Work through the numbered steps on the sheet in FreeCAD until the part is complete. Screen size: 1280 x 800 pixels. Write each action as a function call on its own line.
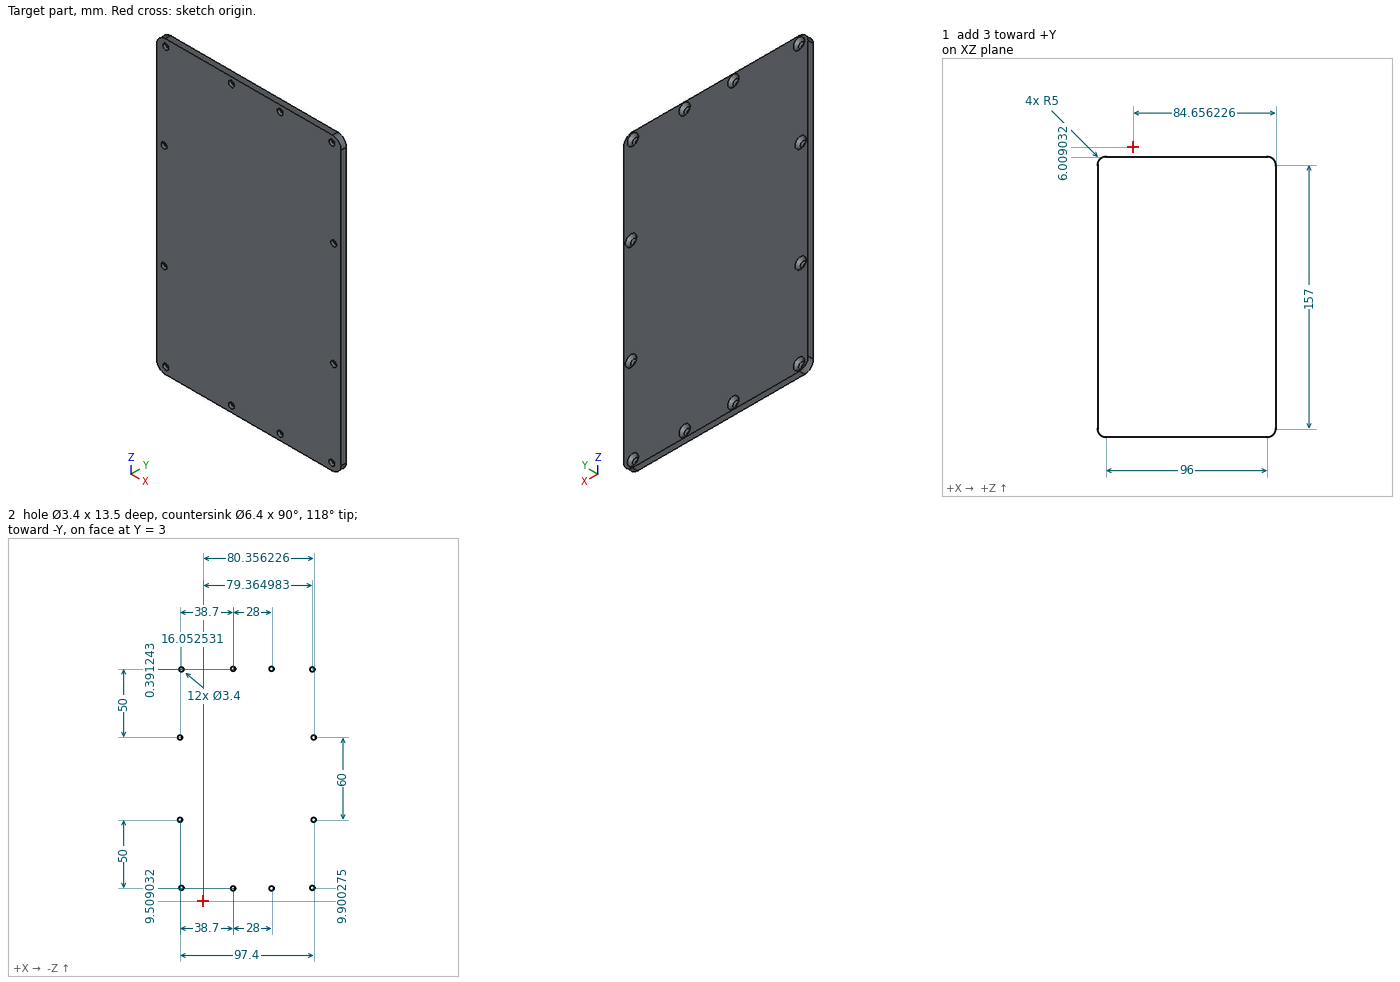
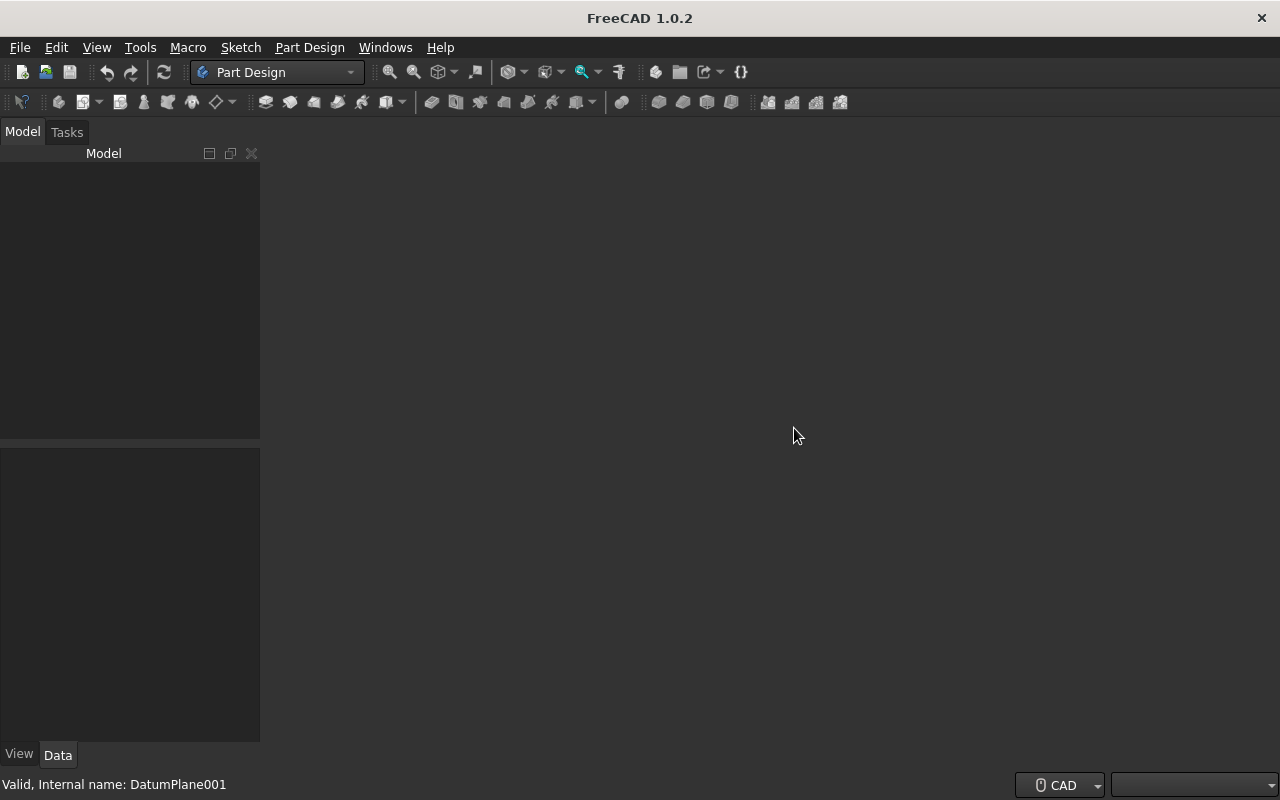
click(22, 72)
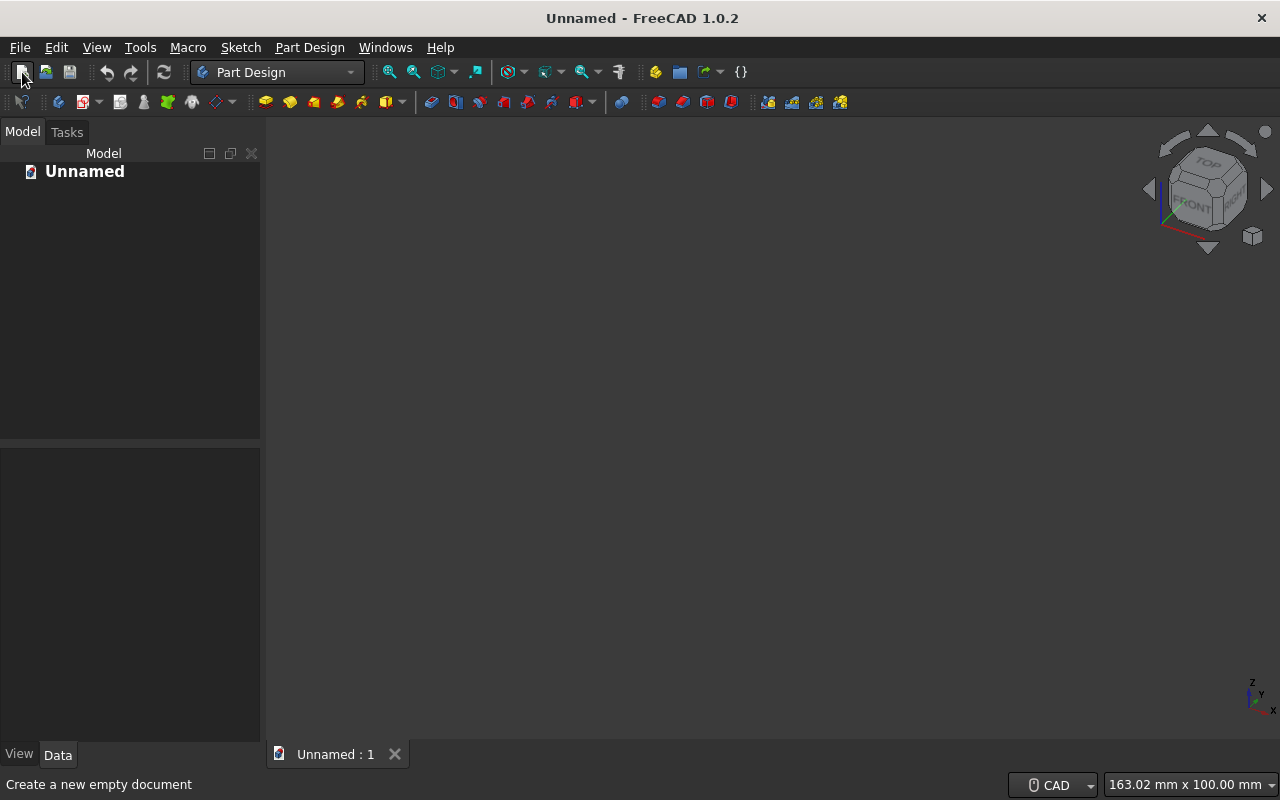
click(84, 102)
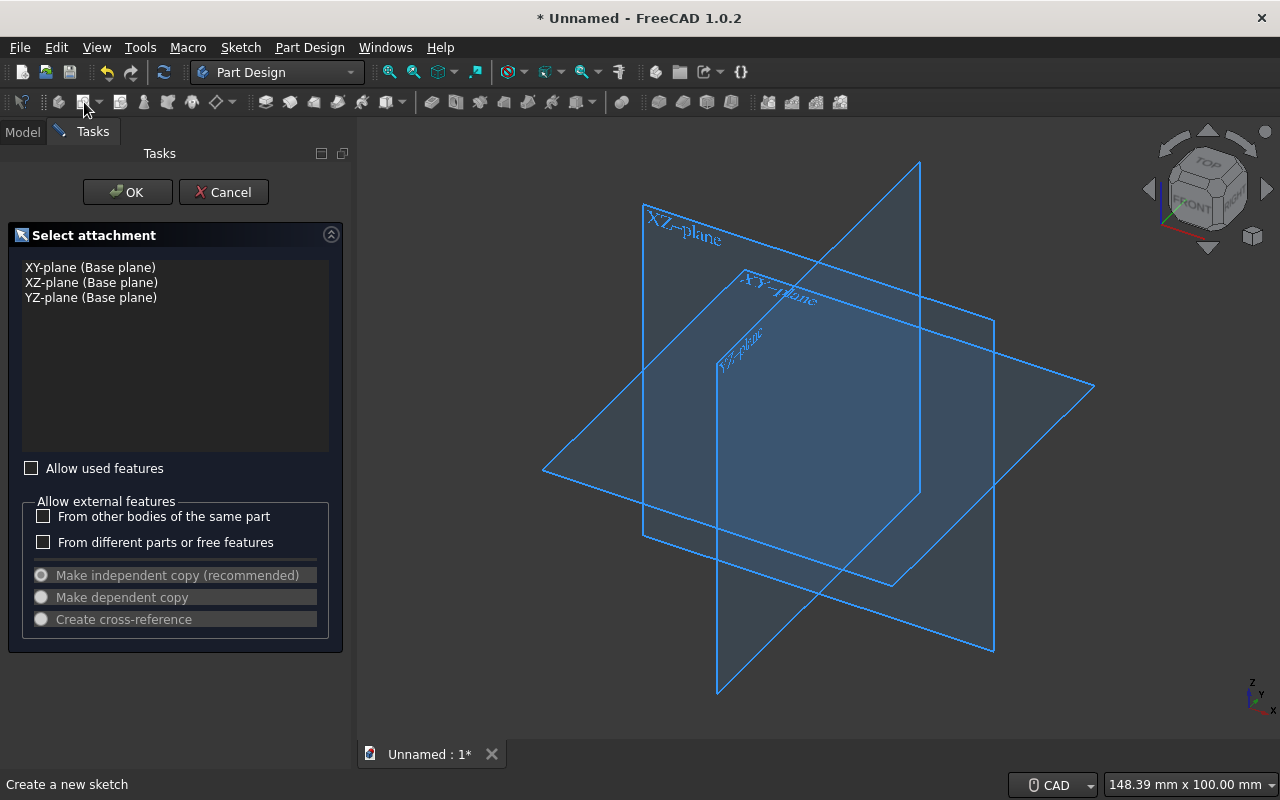
click(82, 282)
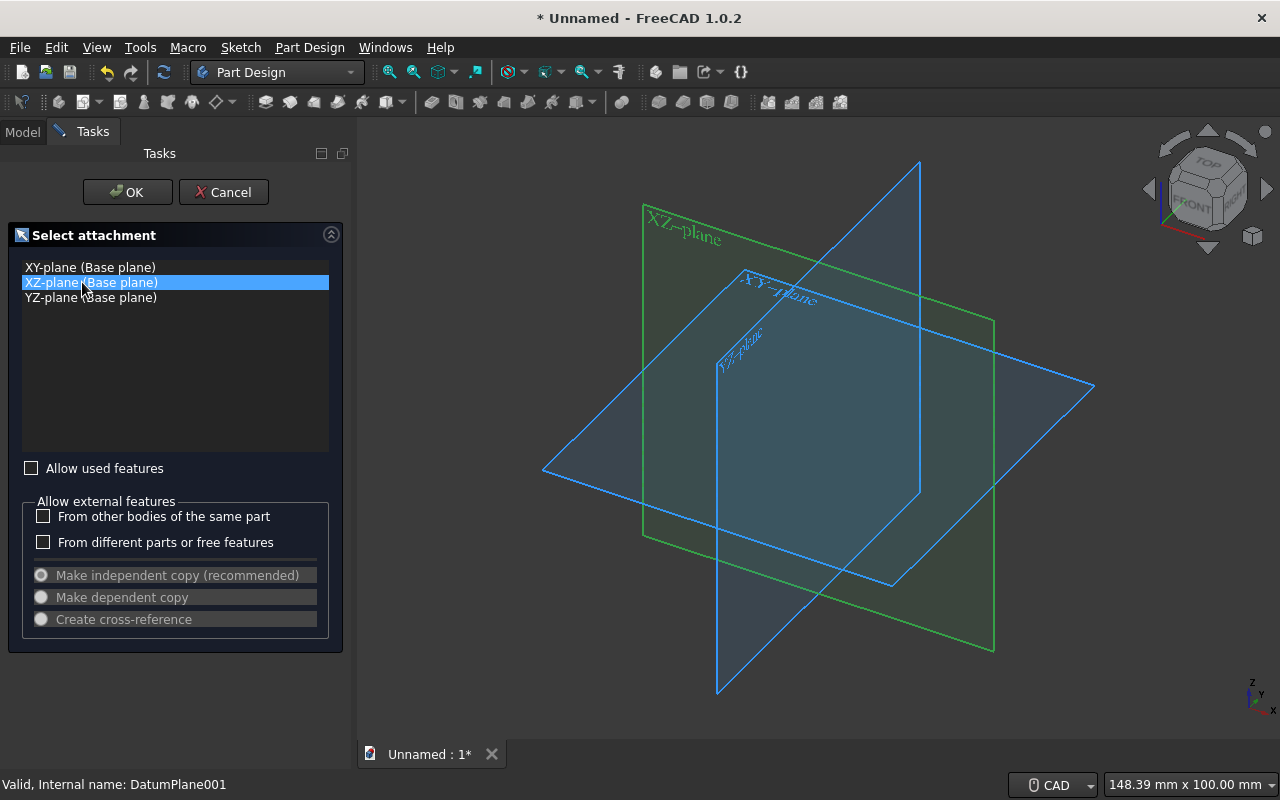
click(128, 192)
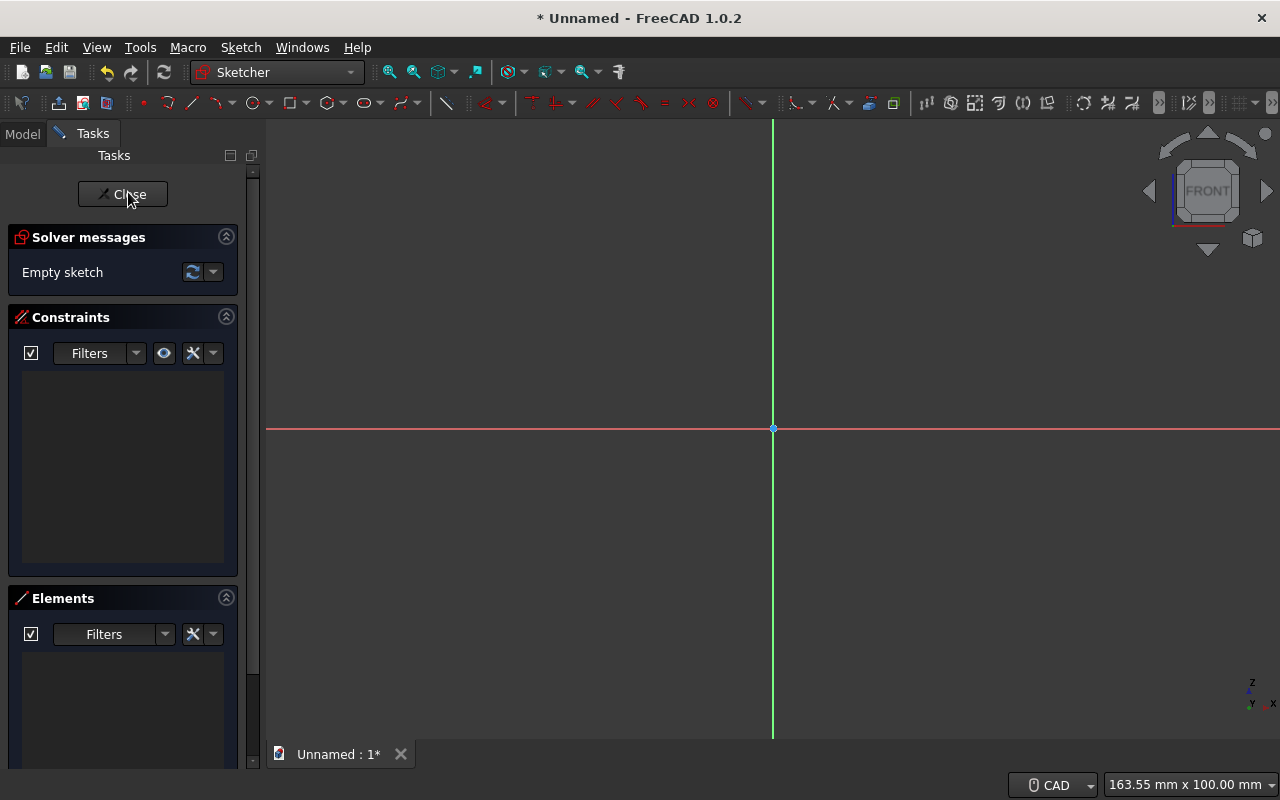
scroll(550, 147, down, 5)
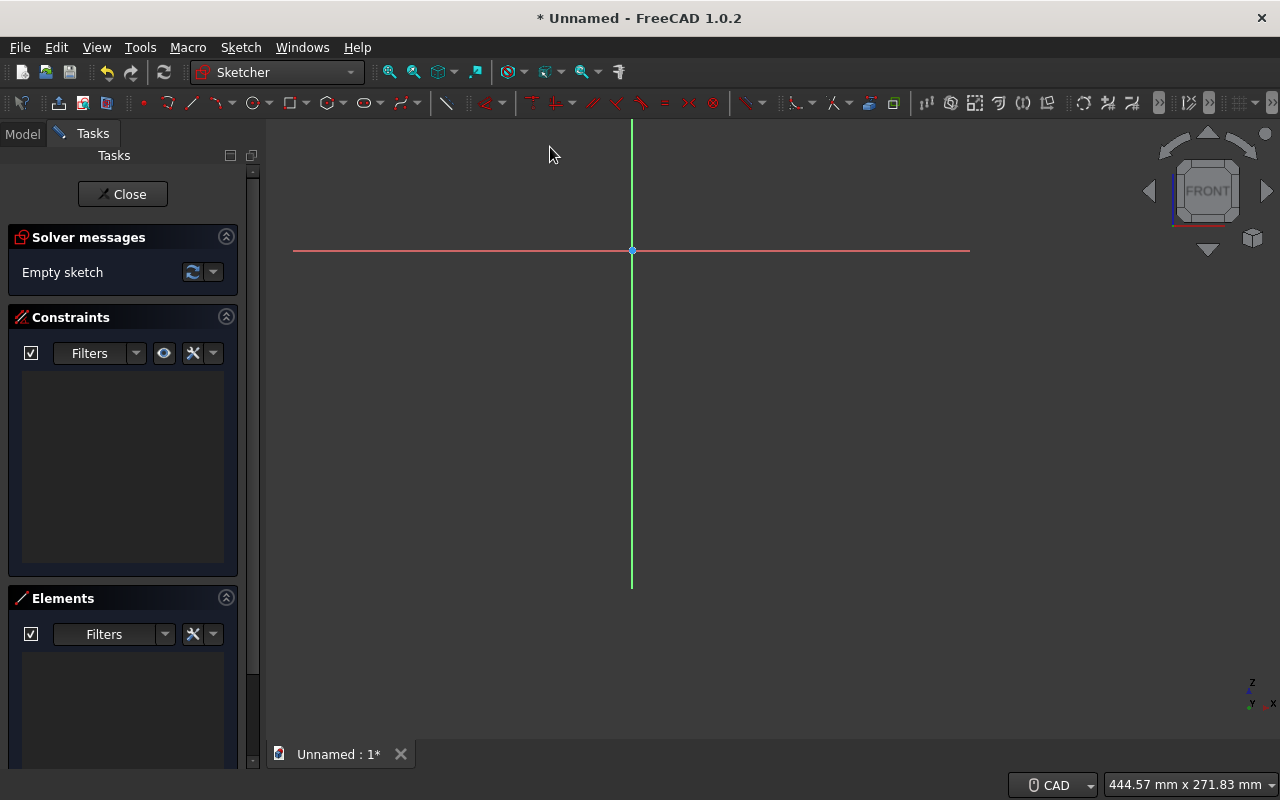
click(192, 104)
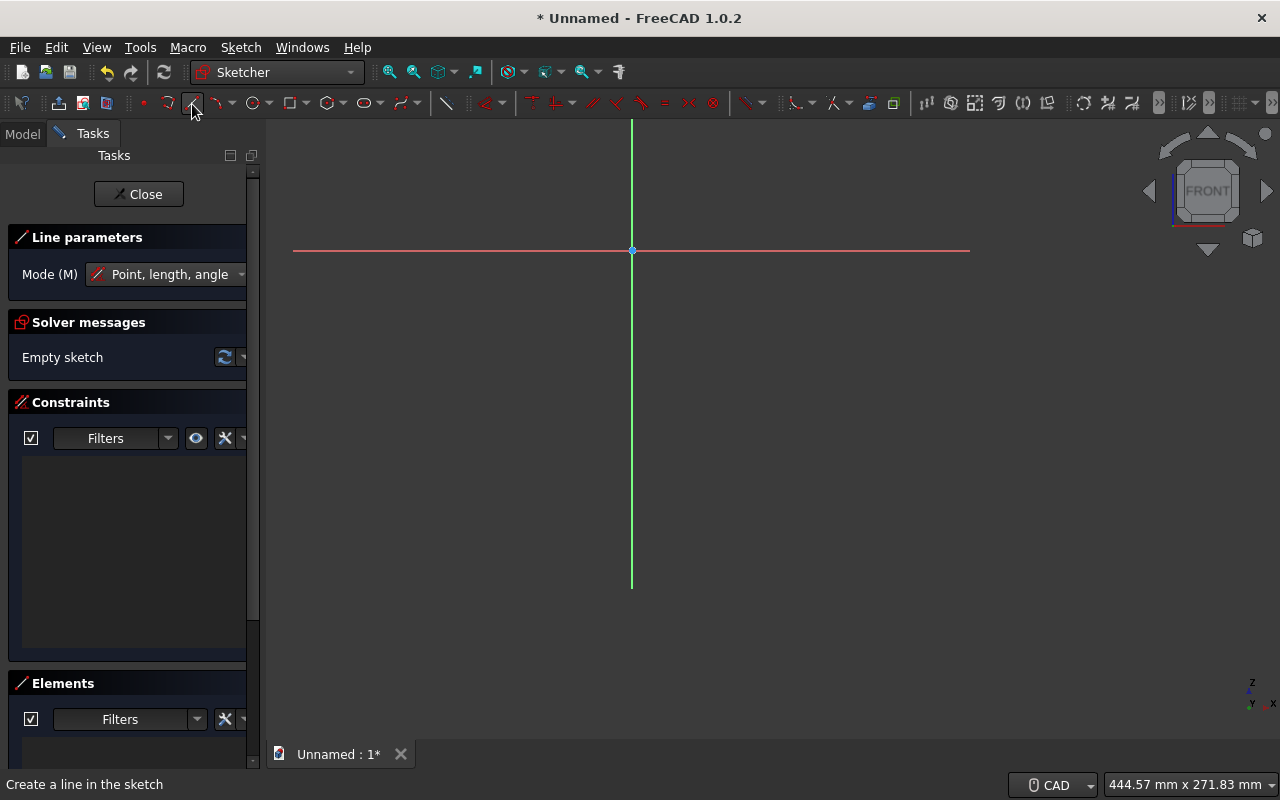
click(825, 276)
click(825, 634)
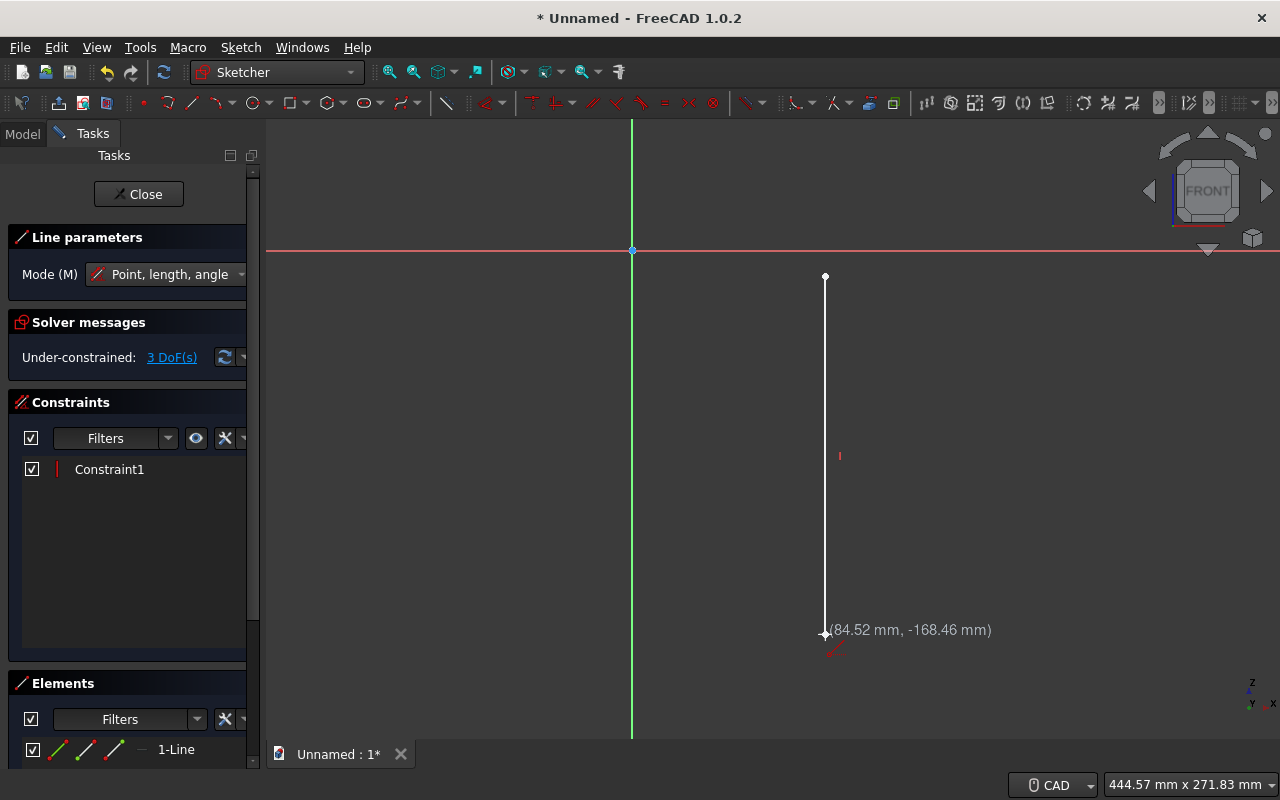
click(814, 645)
click(595, 645)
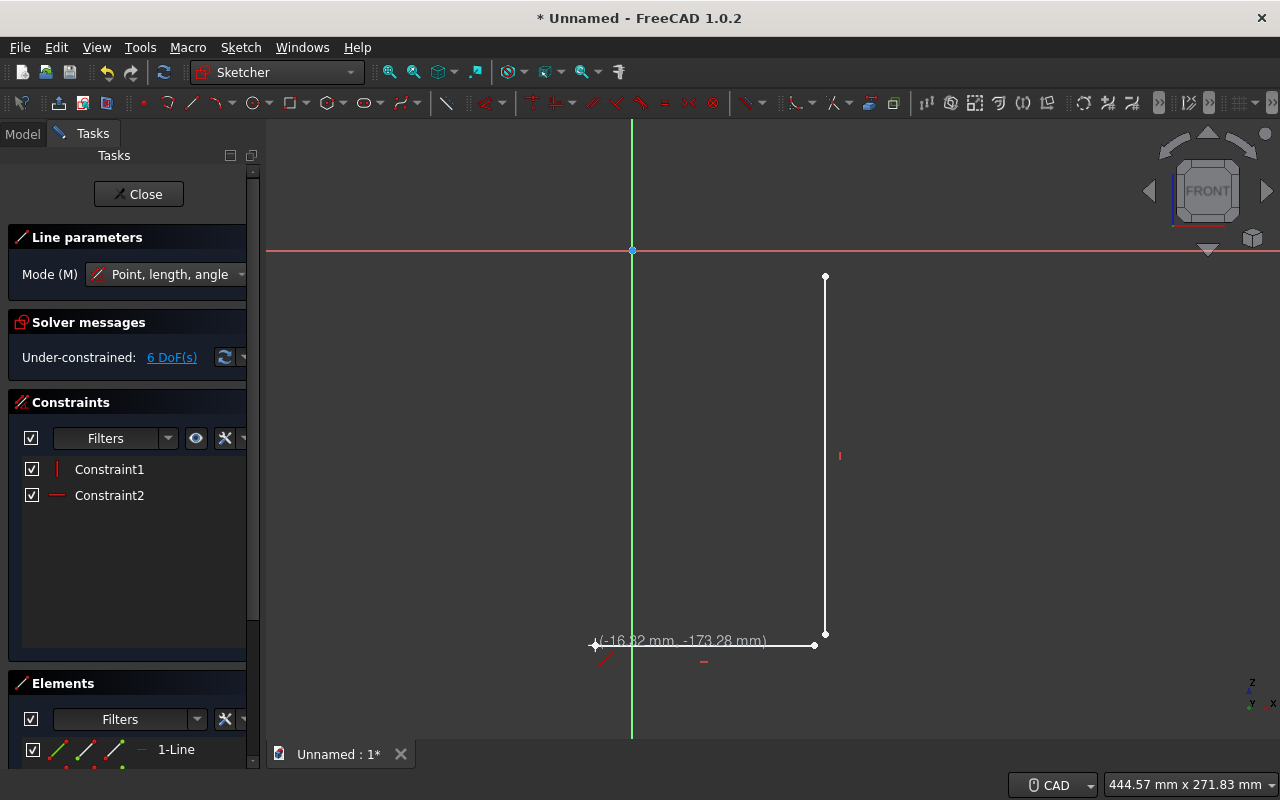
click(584, 634)
click(584, 276)